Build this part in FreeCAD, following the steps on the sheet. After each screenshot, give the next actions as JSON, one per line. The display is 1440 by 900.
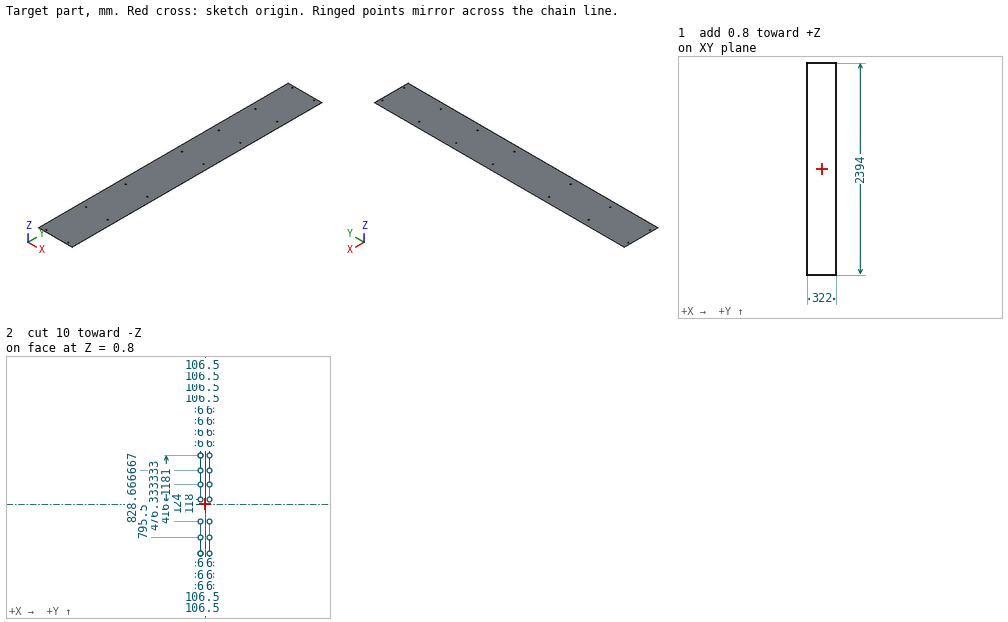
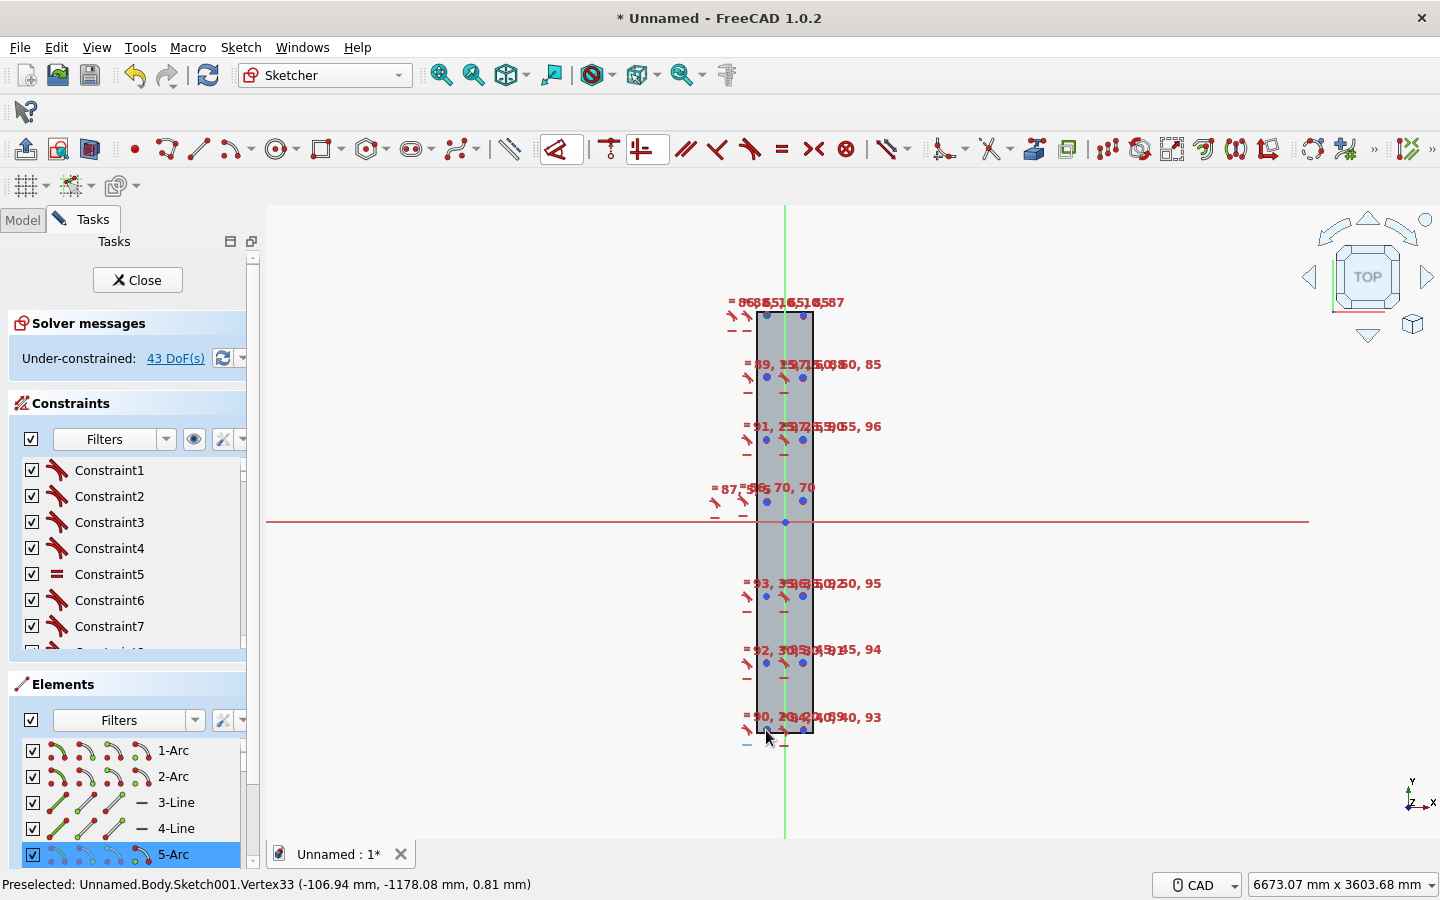
{"action": "left_click", "coordinate": [364, 522]}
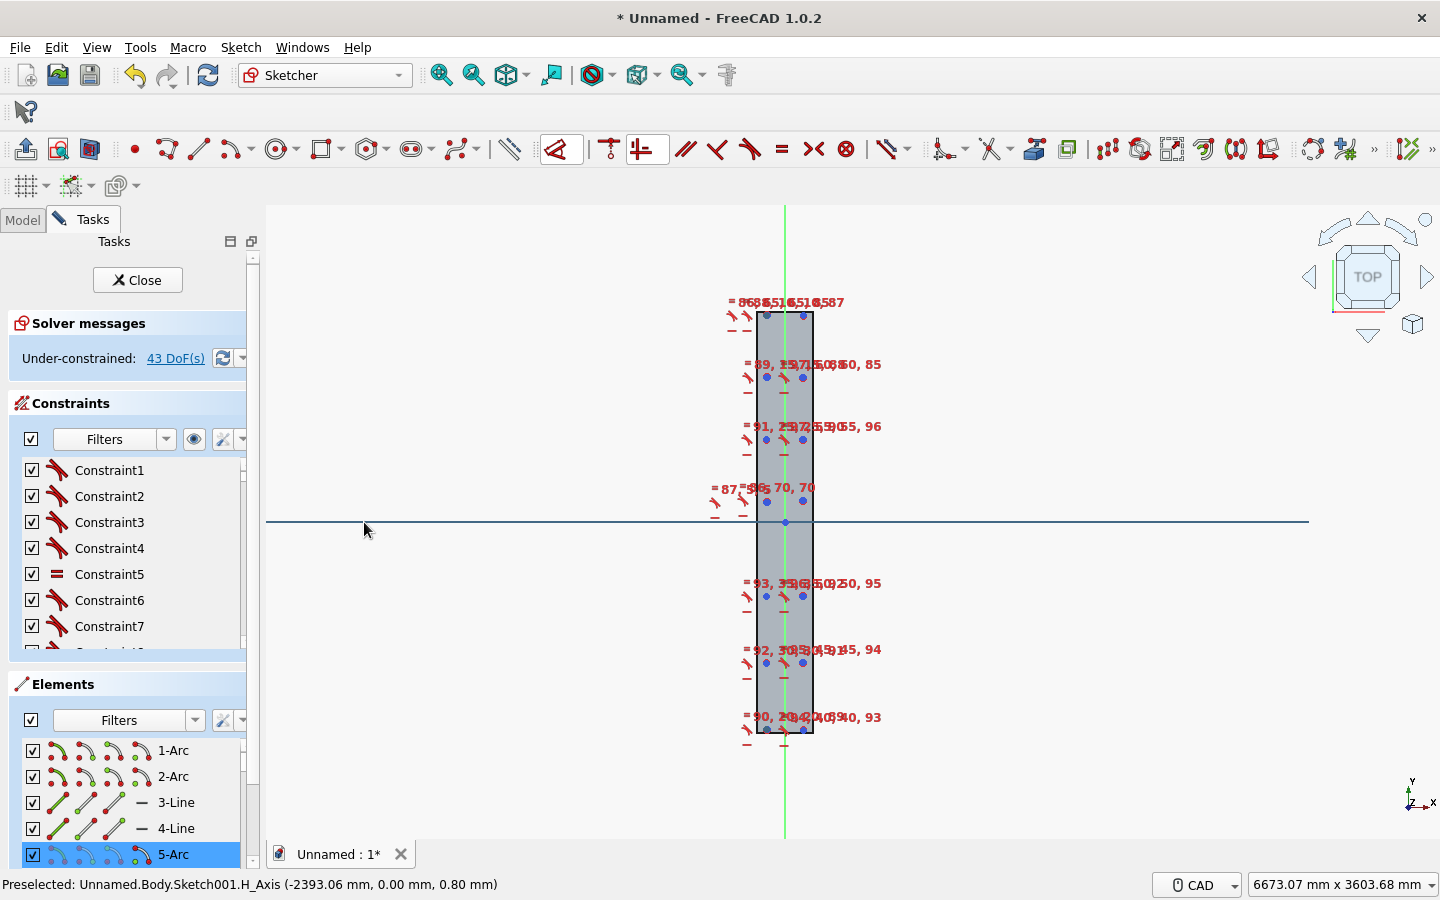
{"action": "key", "text": "s"}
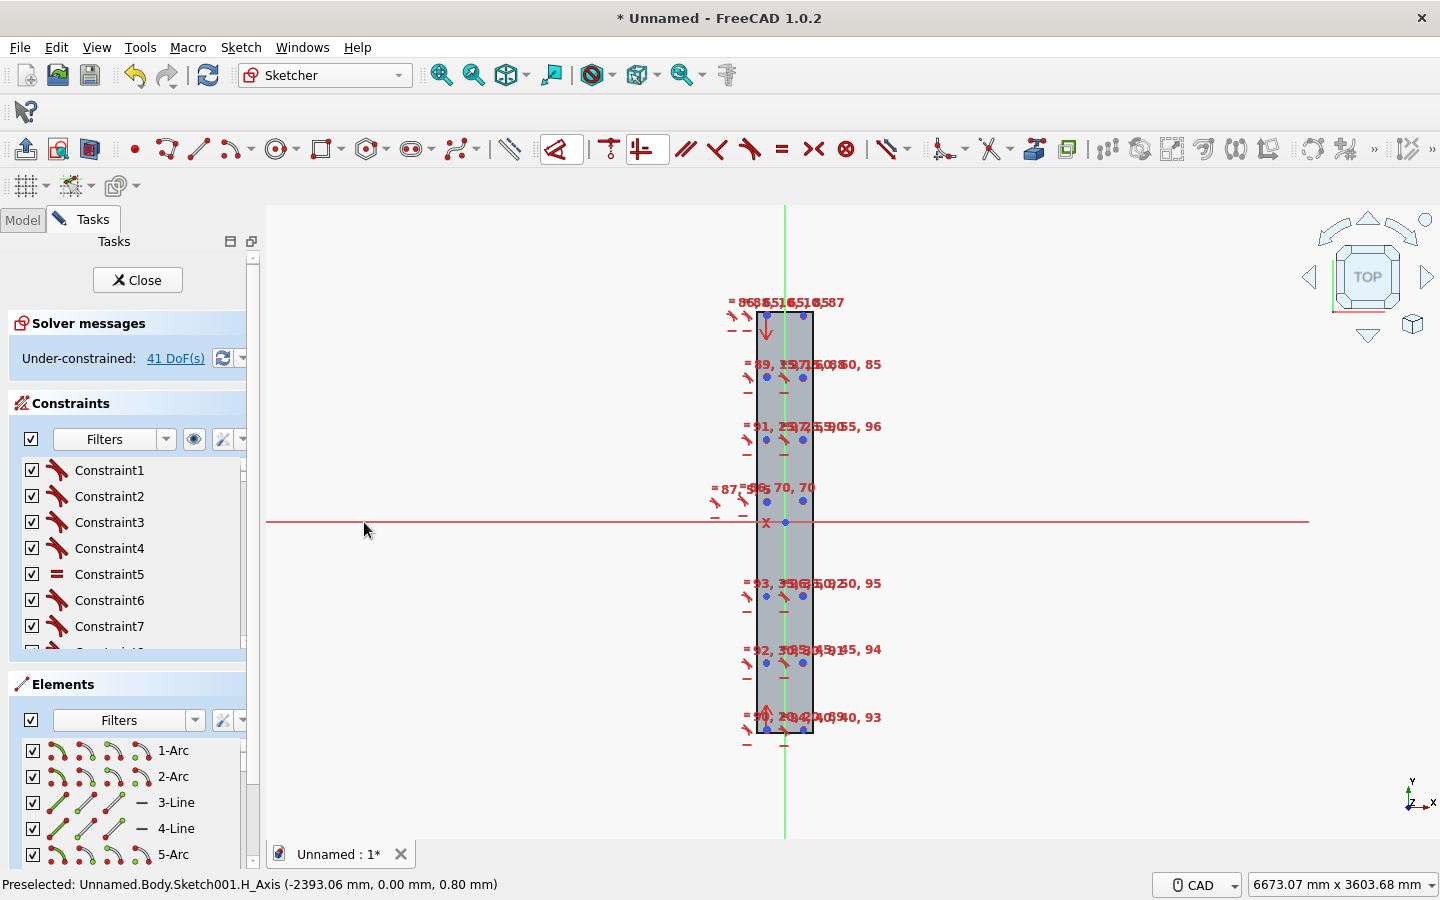
{"action": "scroll", "coordinate": [767, 730], "scroll_direction": "up", "scroll_amount": 14}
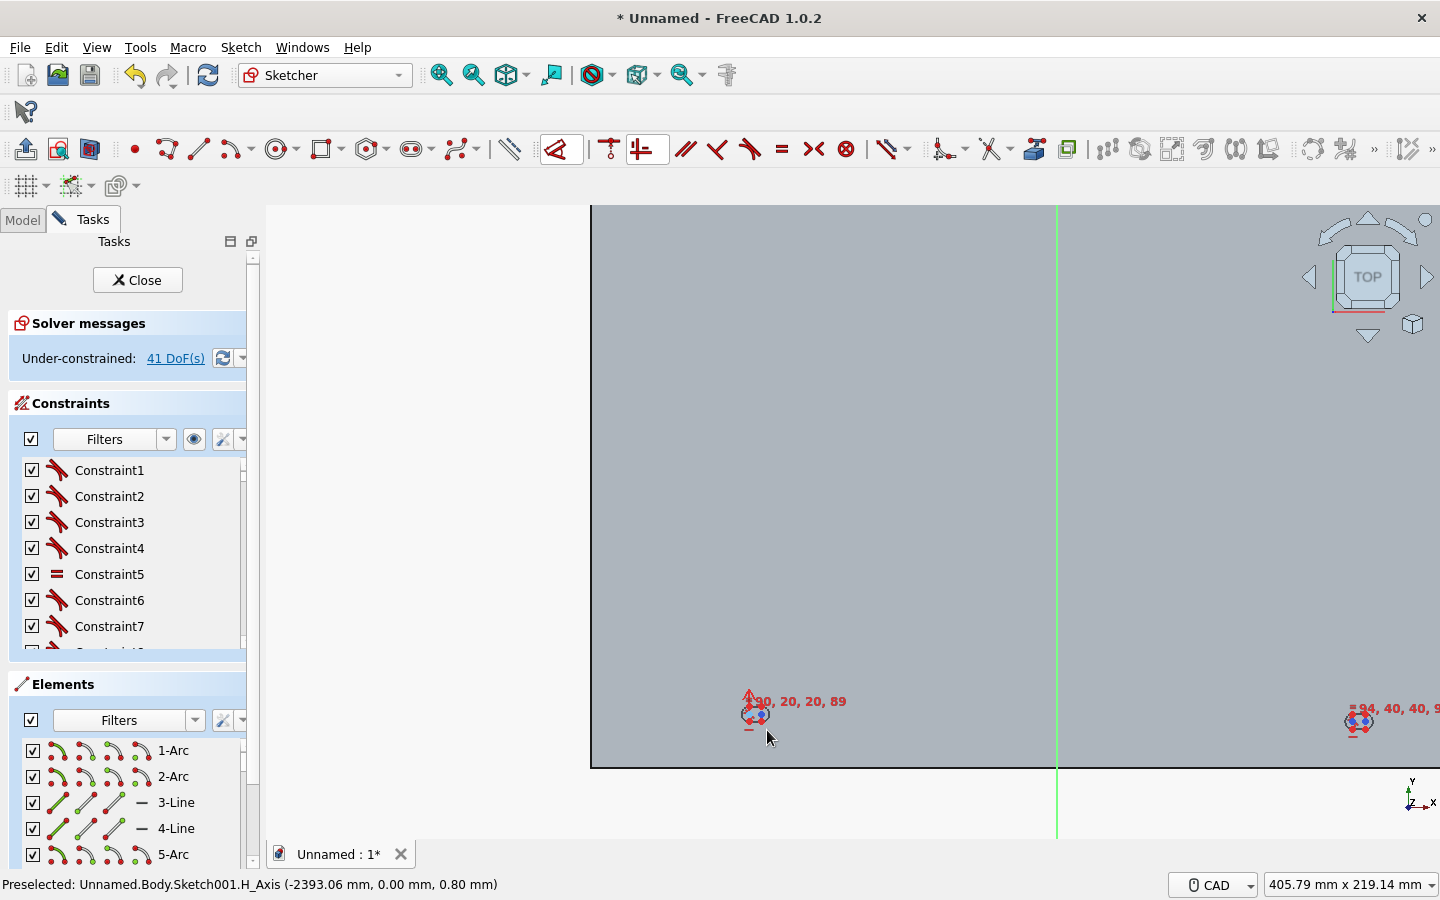
{"action": "left_click", "coordinate": [762, 714]}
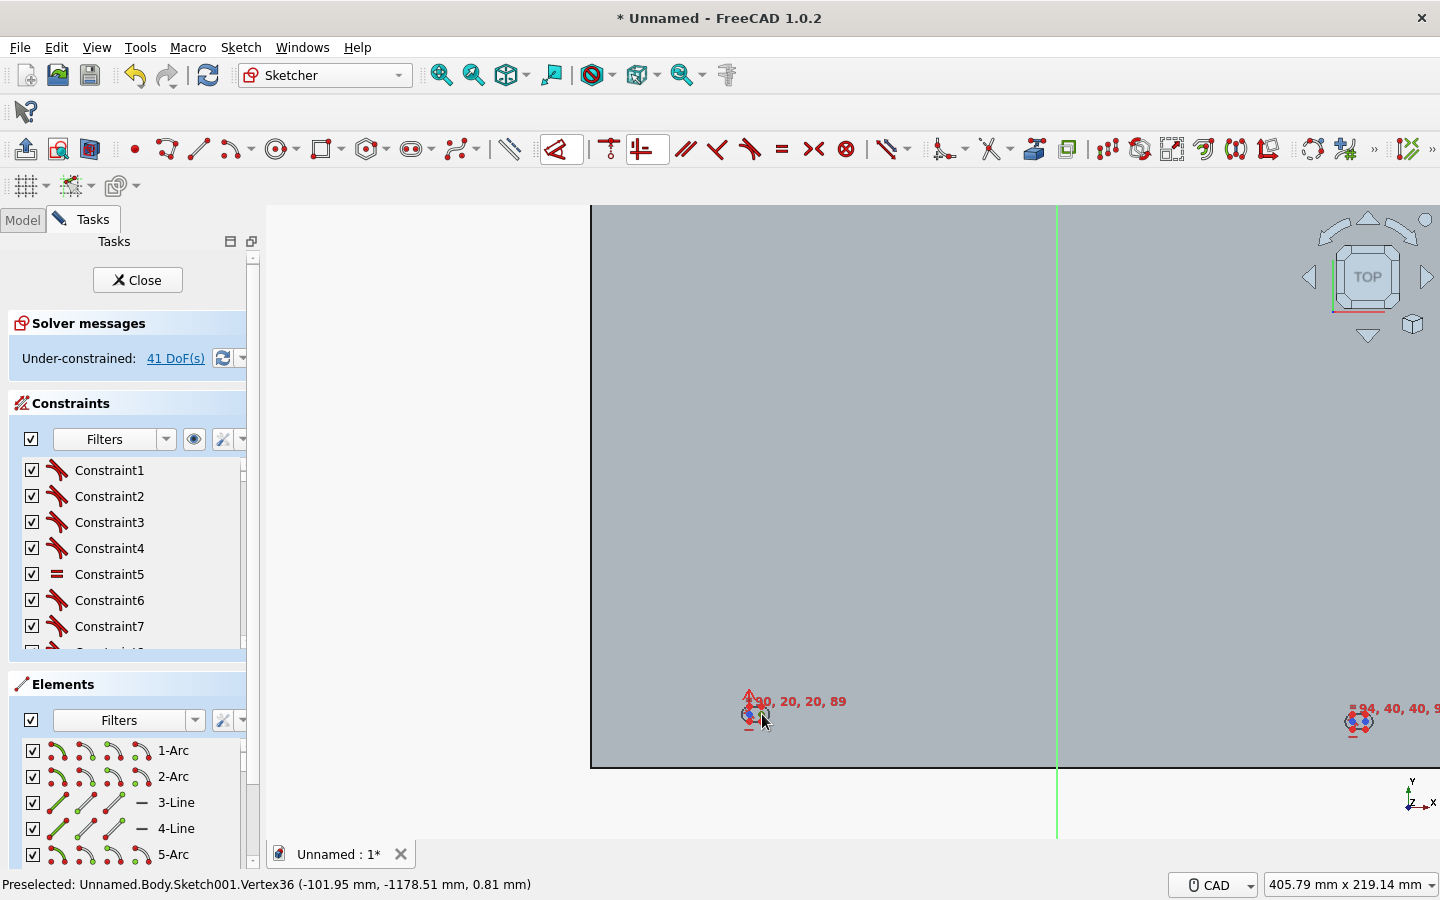
{"action": "scroll", "coordinate": [767, 730], "scroll_direction": "down", "scroll_amount": 14}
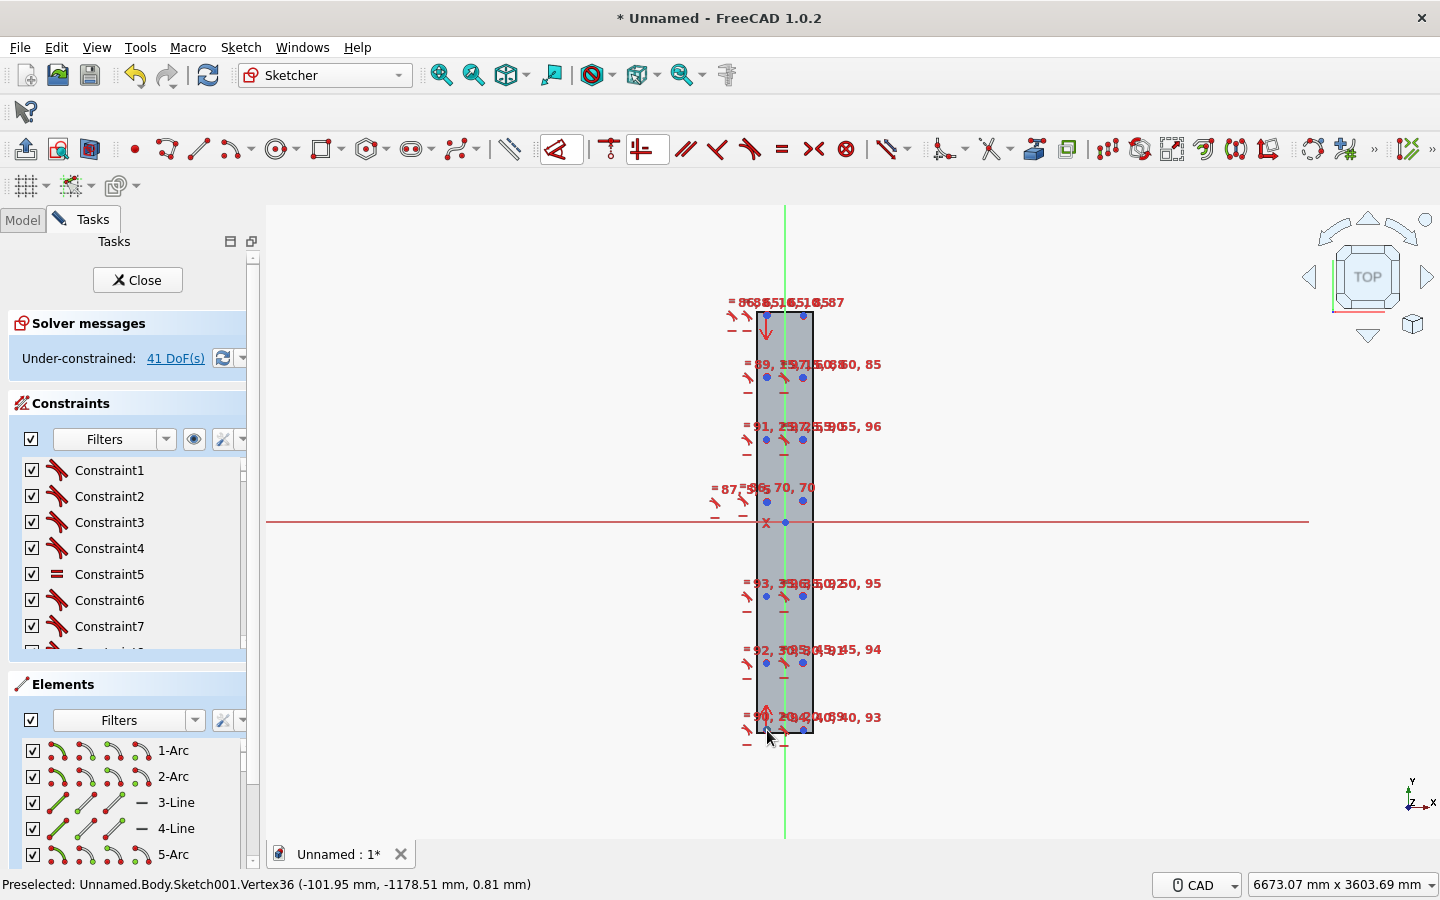
{"action": "scroll", "coordinate": [803, 730], "scroll_direction": "up", "scroll_amount": 14}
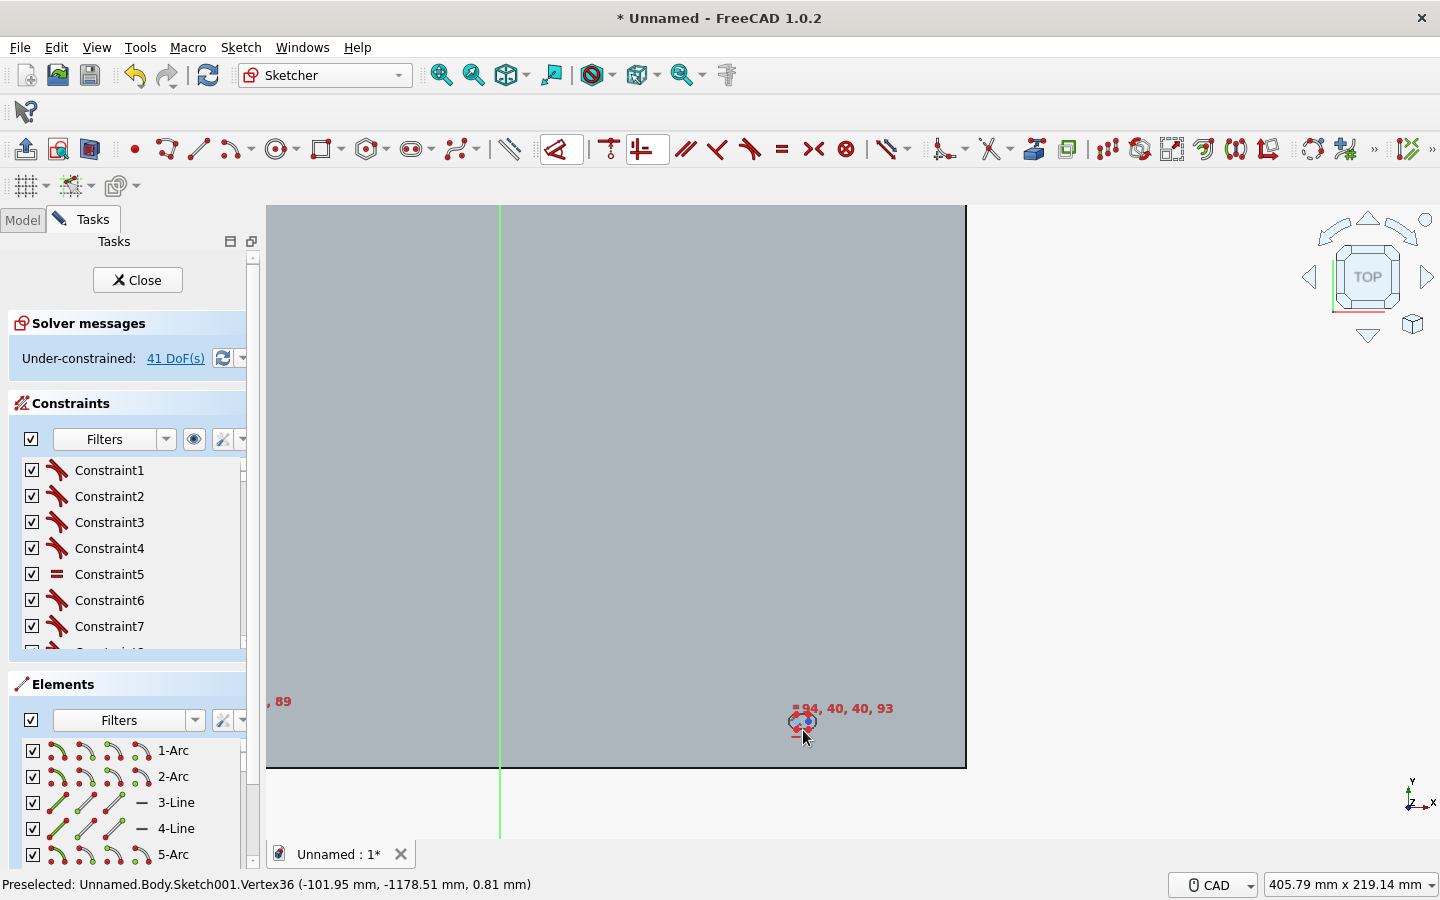
{"action": "left_click", "coordinate": [796, 722]}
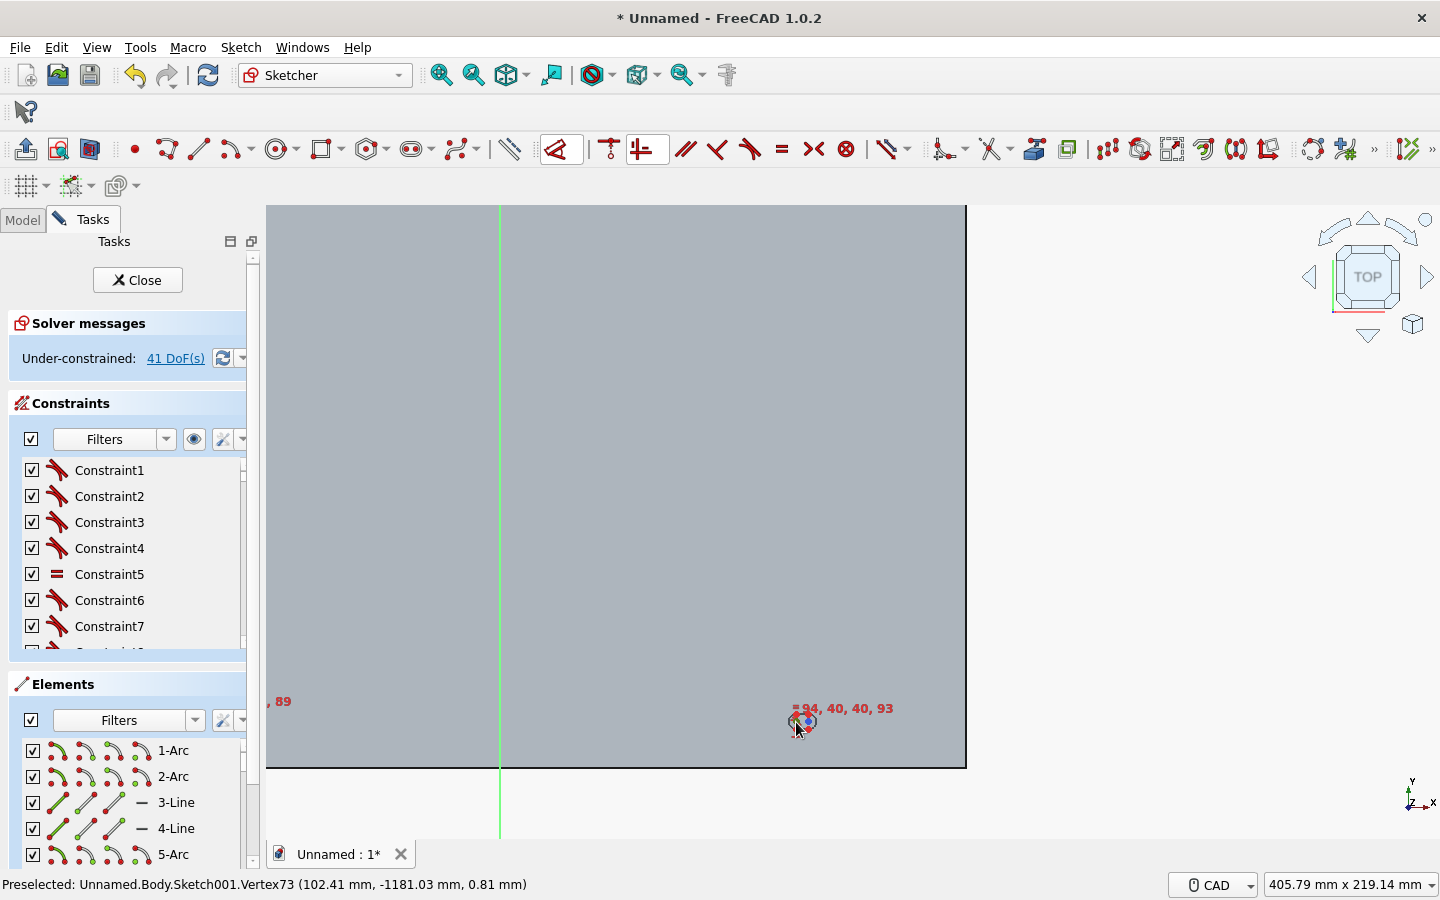
{"action": "left_click", "coordinate": [500, 770]}